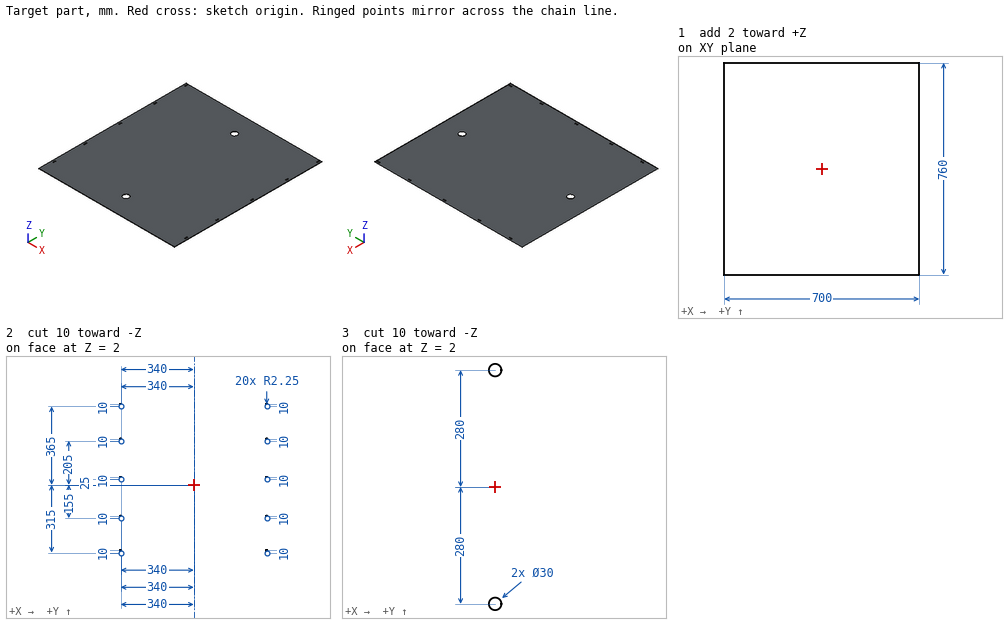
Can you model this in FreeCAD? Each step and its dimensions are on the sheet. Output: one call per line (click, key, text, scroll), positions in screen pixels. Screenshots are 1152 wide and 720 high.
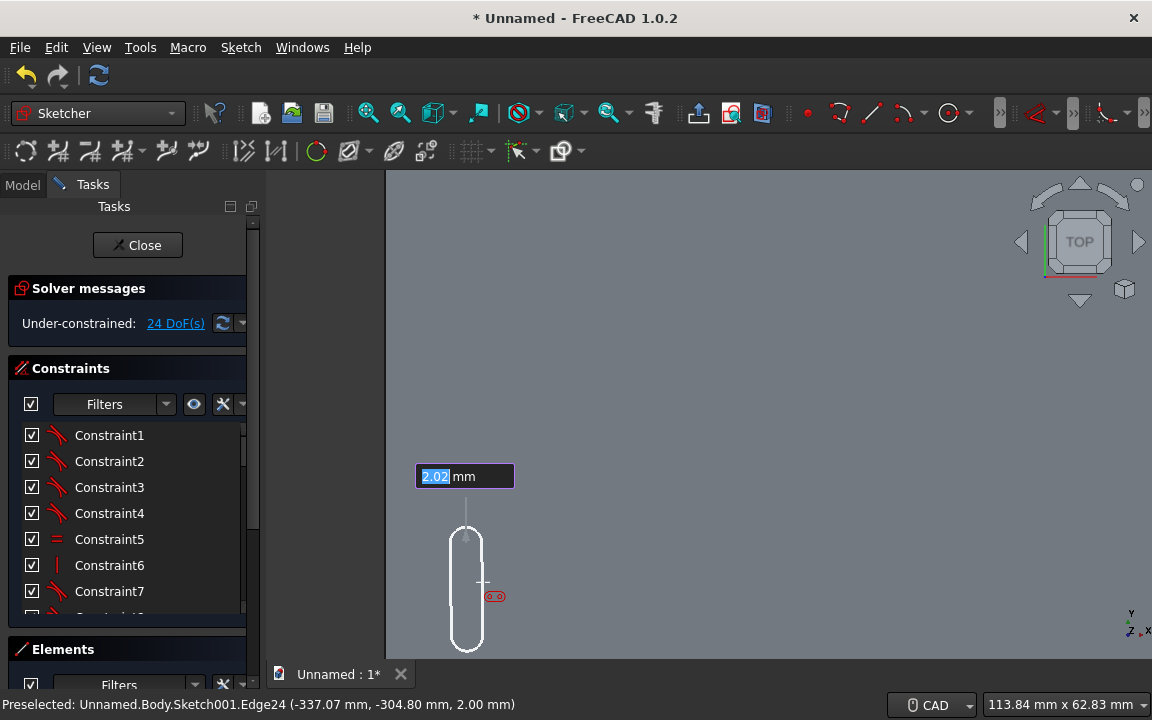
click(481, 579)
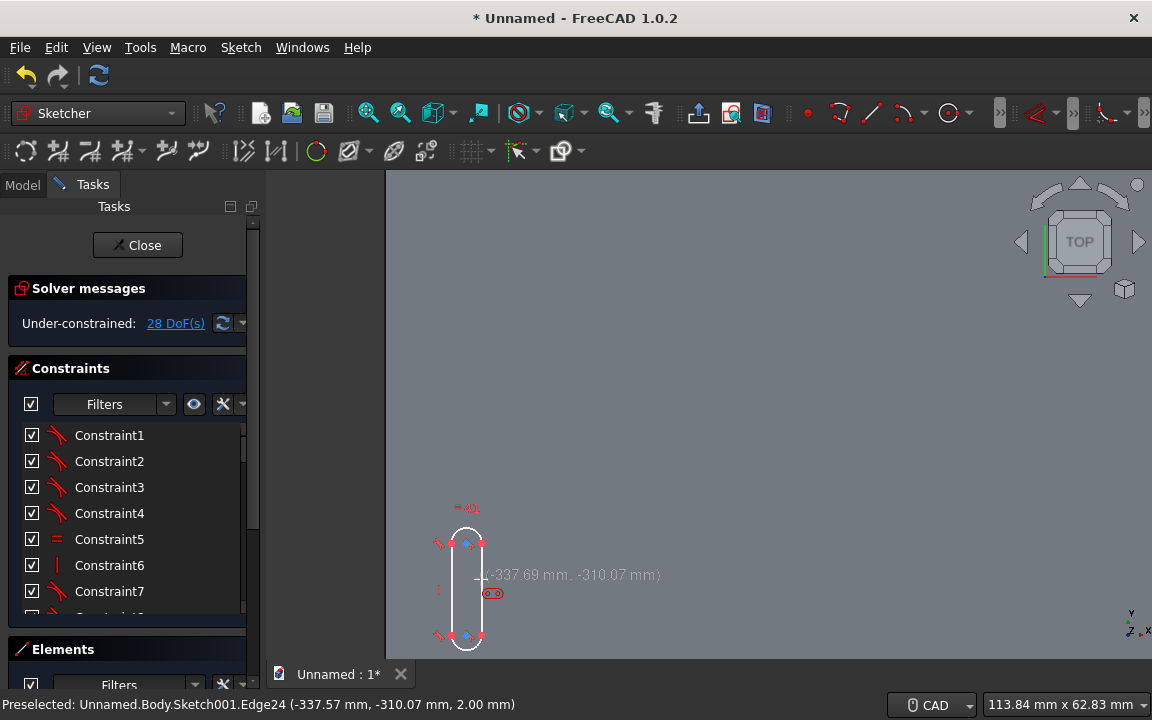
scroll(481, 575, down, 14)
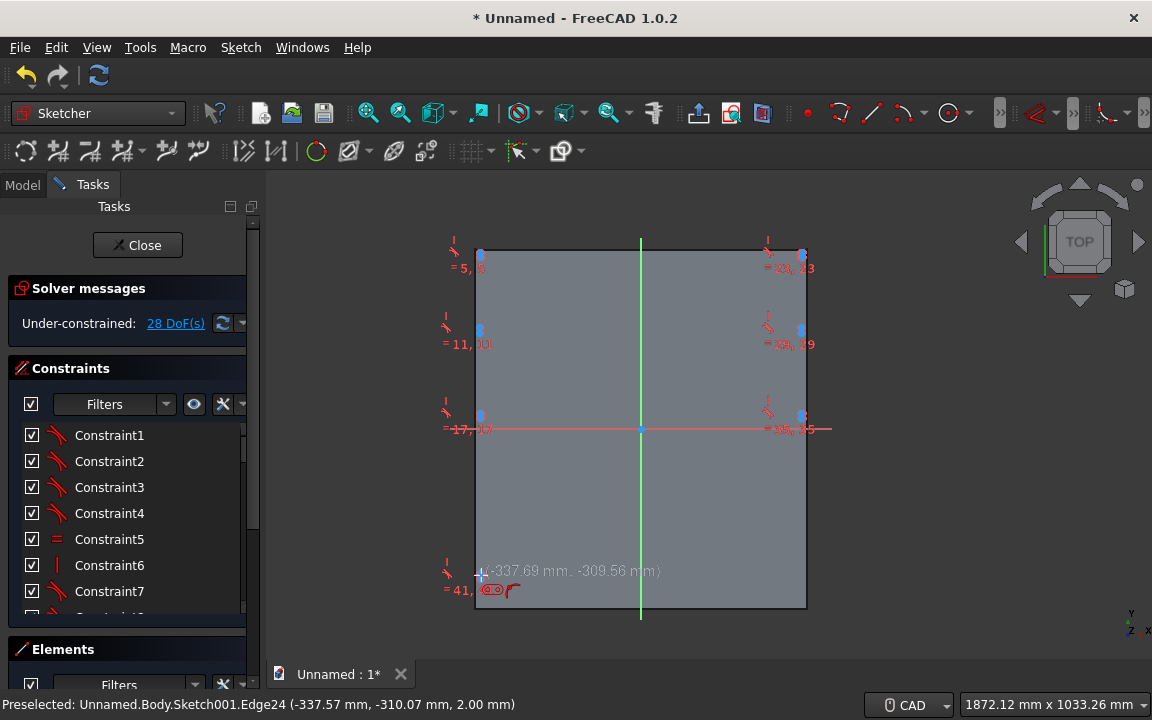
scroll(480, 503, up, 16)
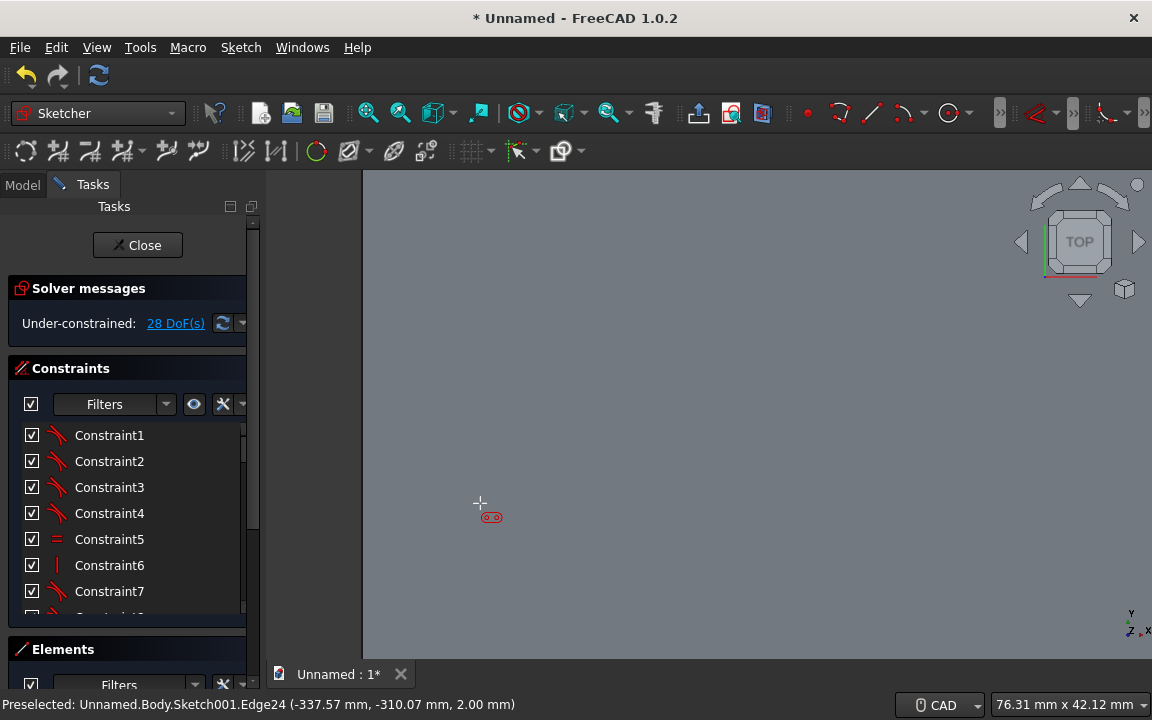
scroll(480, 503, down, 16)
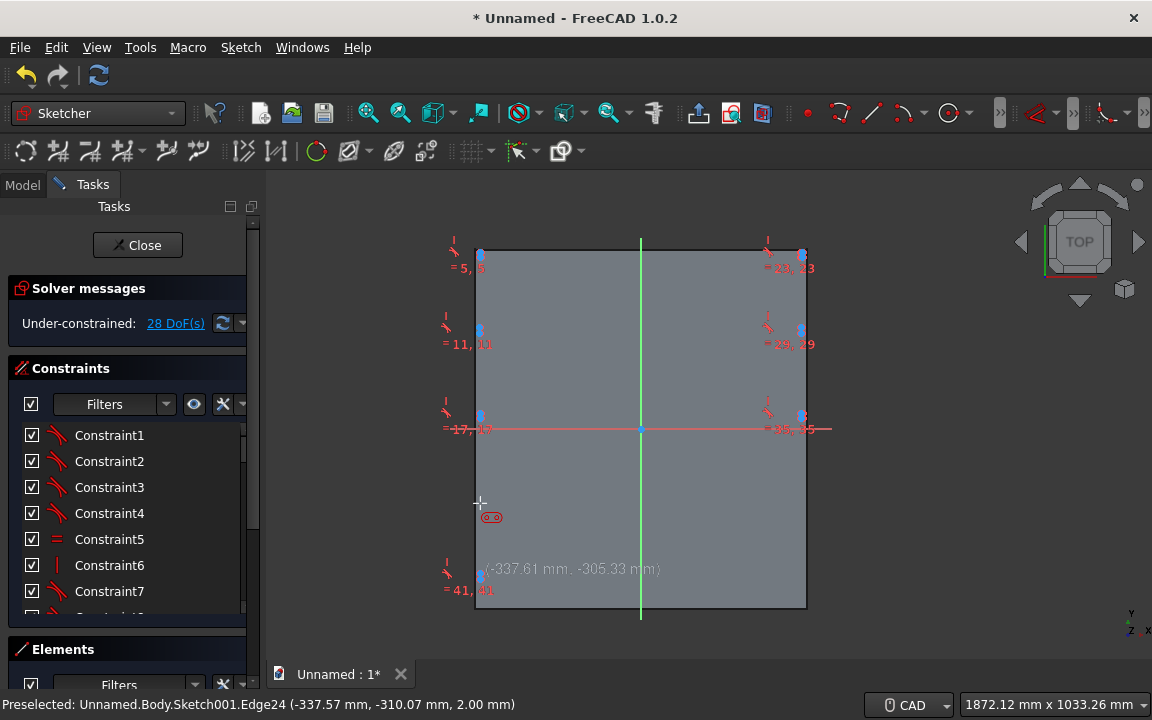
click(480, 503)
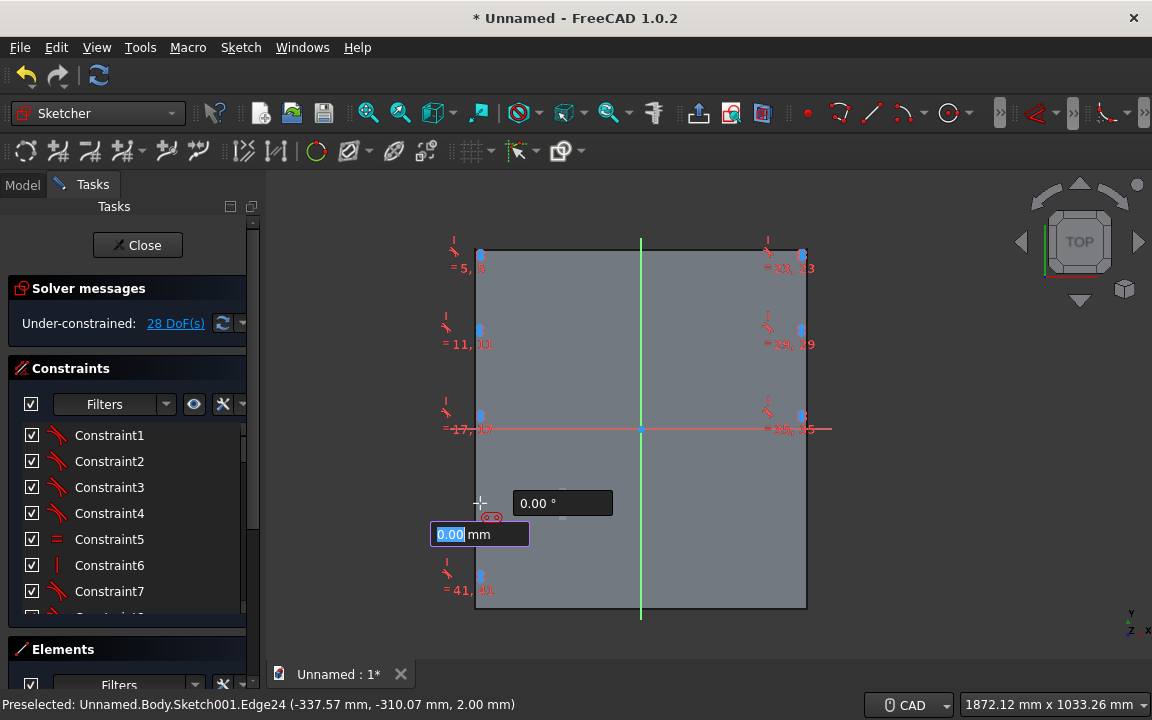
scroll(480, 498, up, 7)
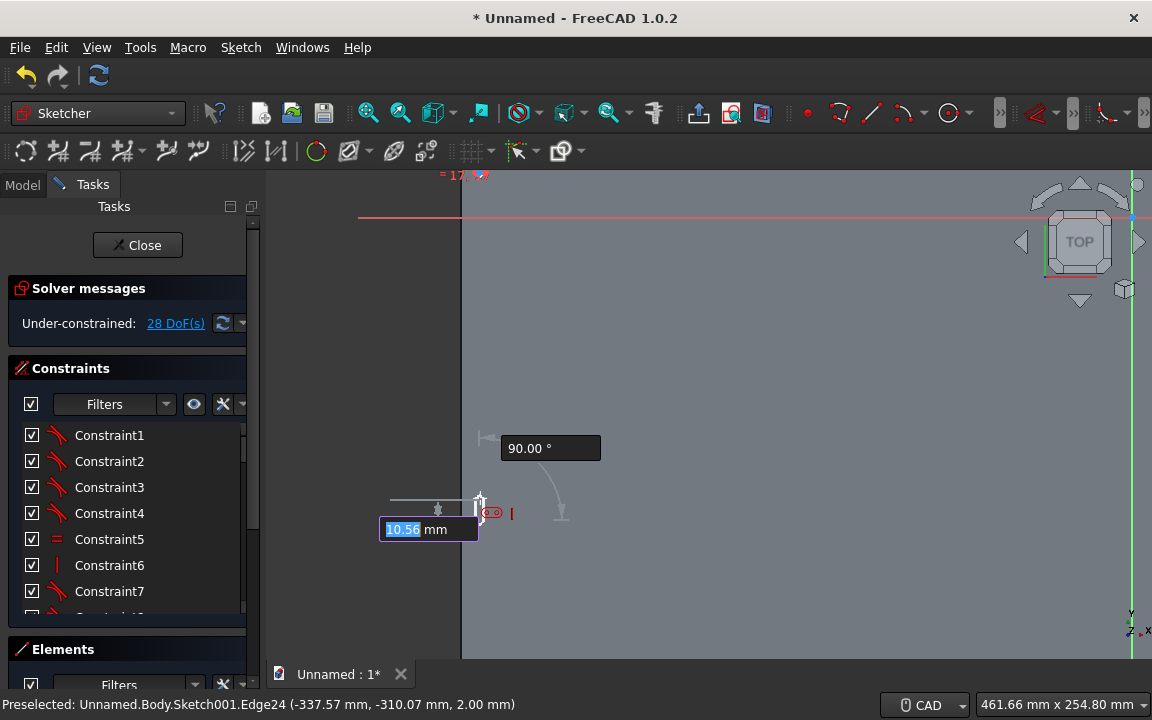
click(479, 496)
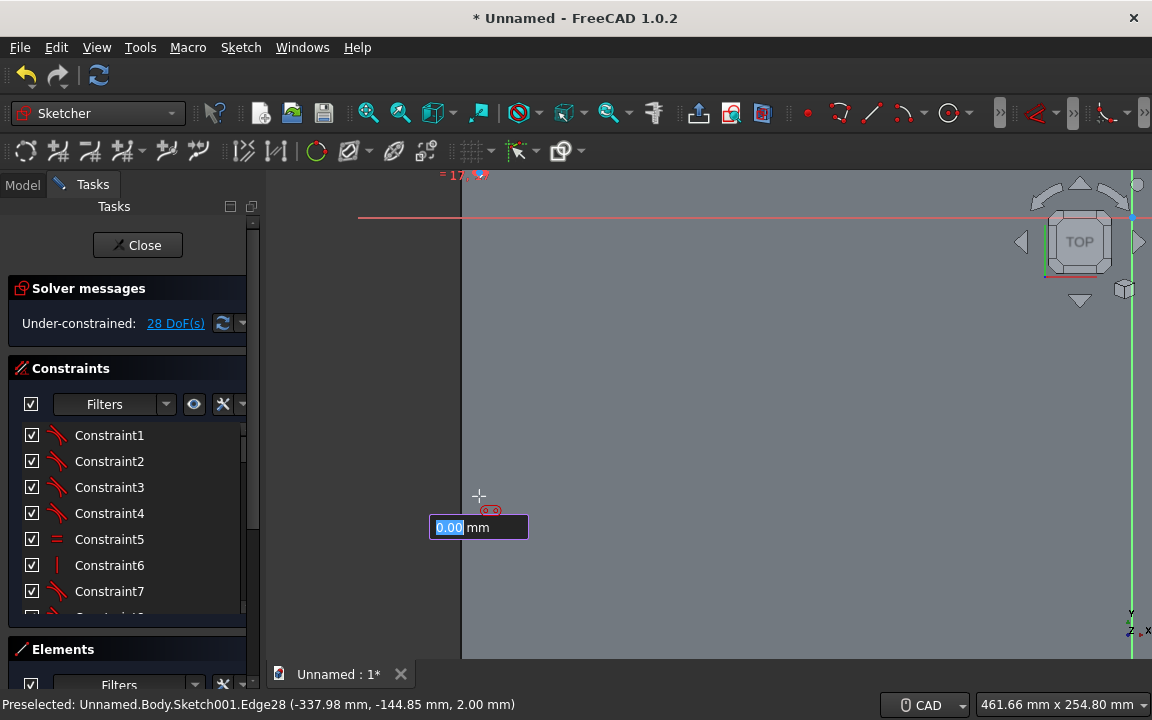
scroll(484, 505, up, 7)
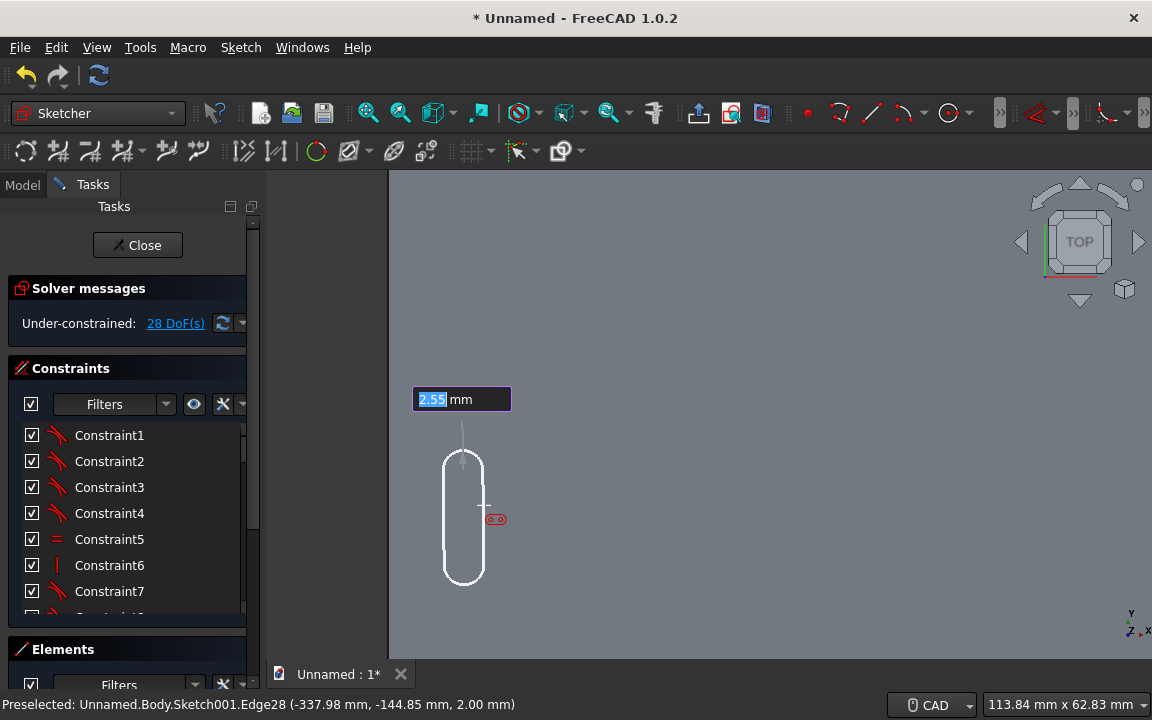
click(484, 504)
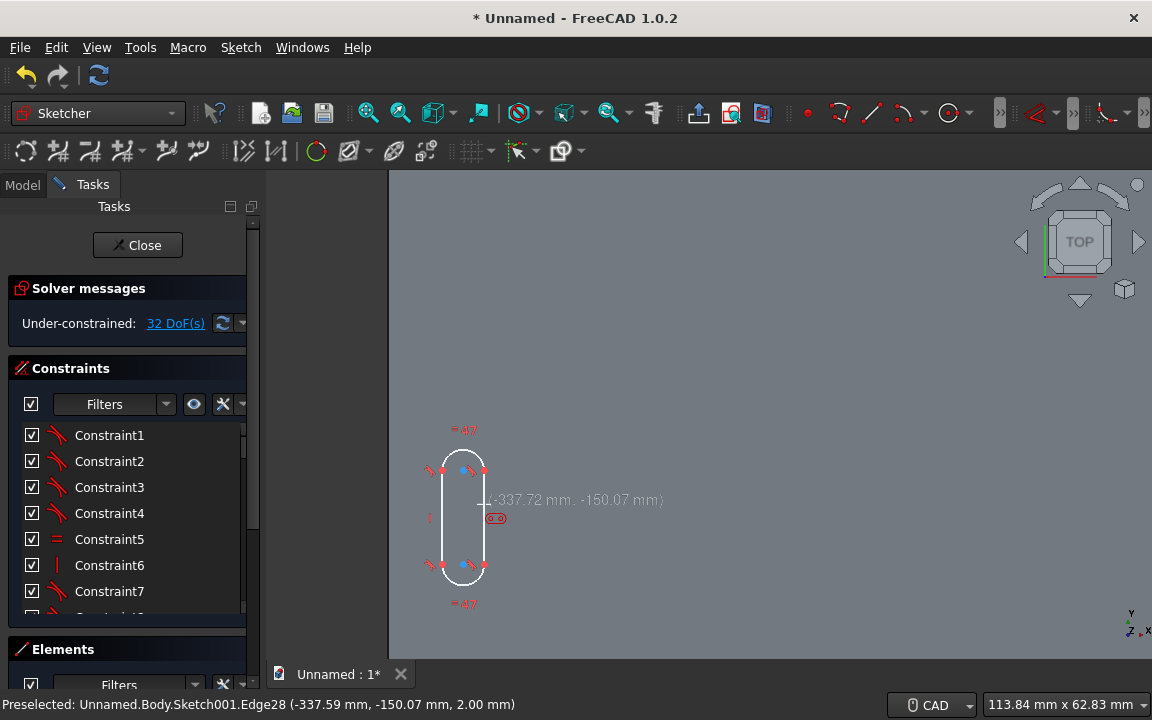
scroll(480, 499, down, 14)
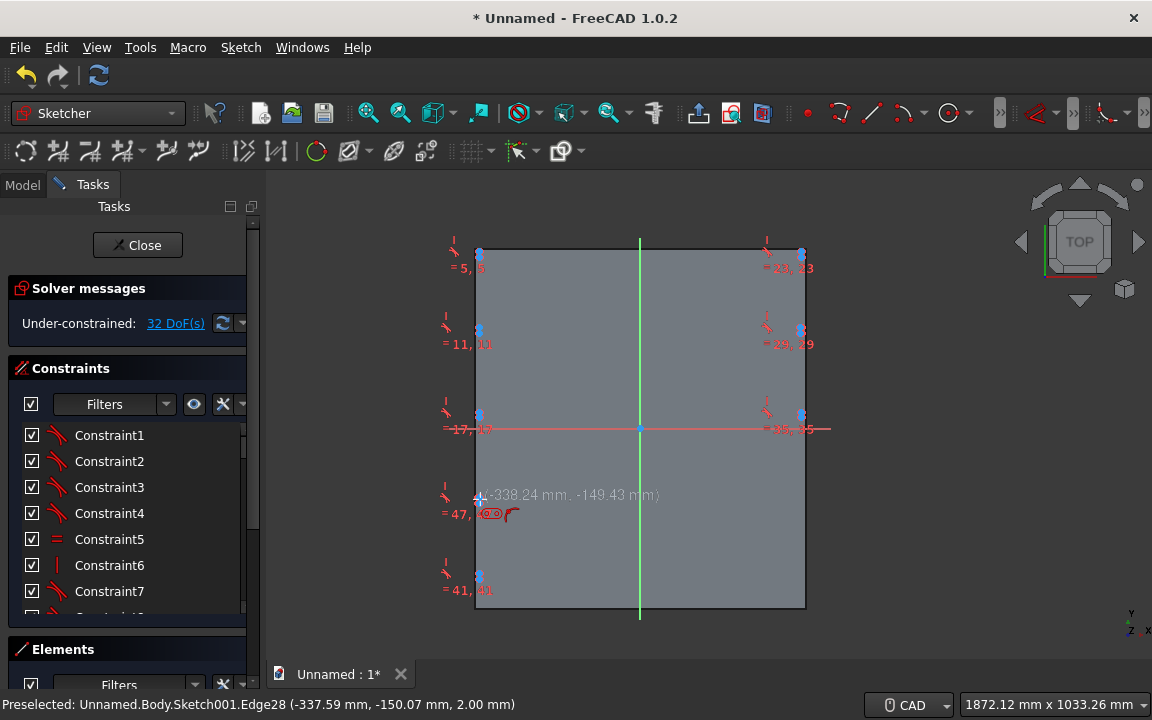
scroll(801, 578, up, 16)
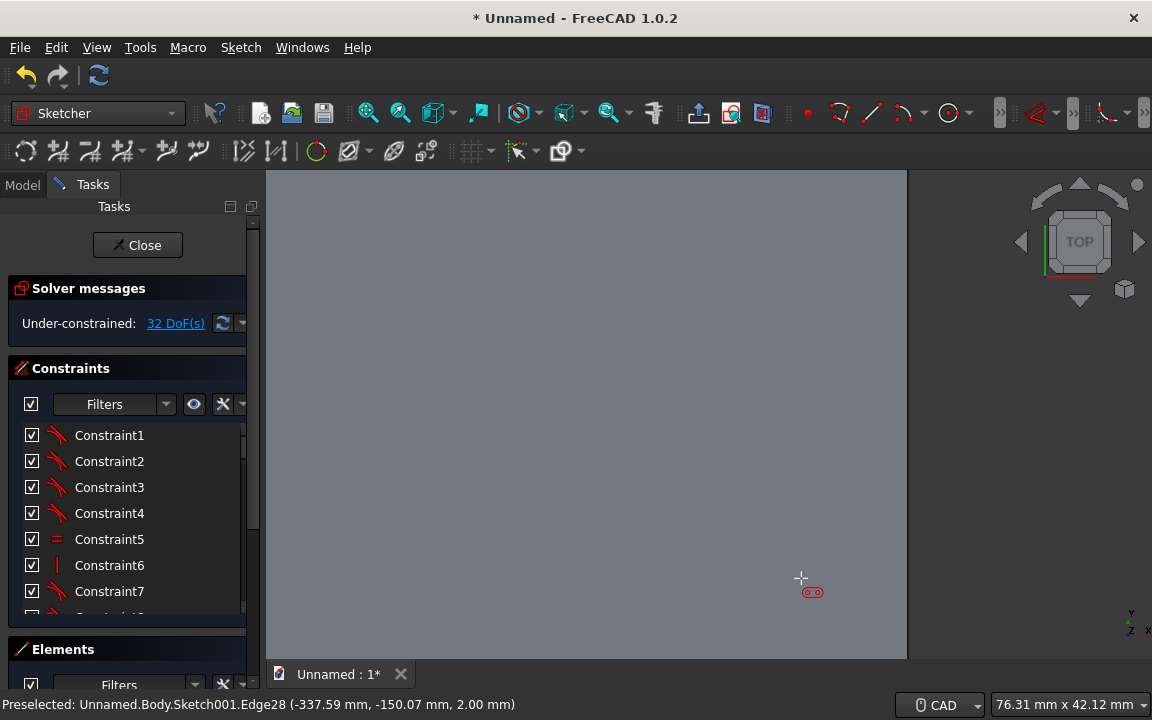
scroll(802, 579, down, 16)